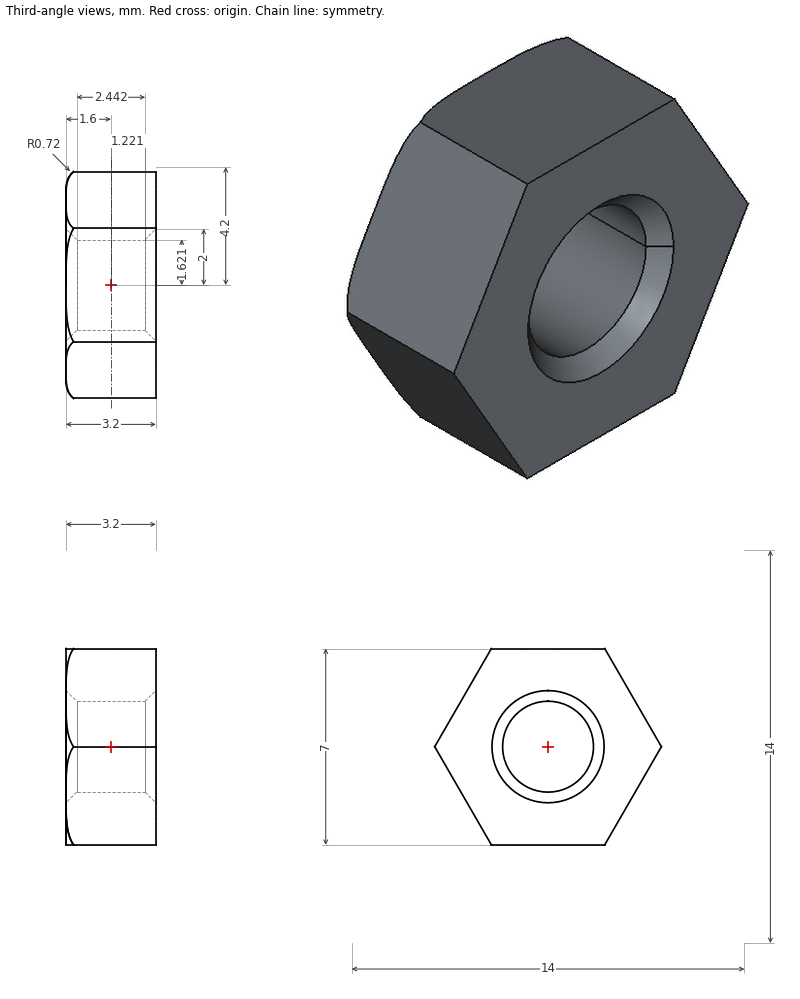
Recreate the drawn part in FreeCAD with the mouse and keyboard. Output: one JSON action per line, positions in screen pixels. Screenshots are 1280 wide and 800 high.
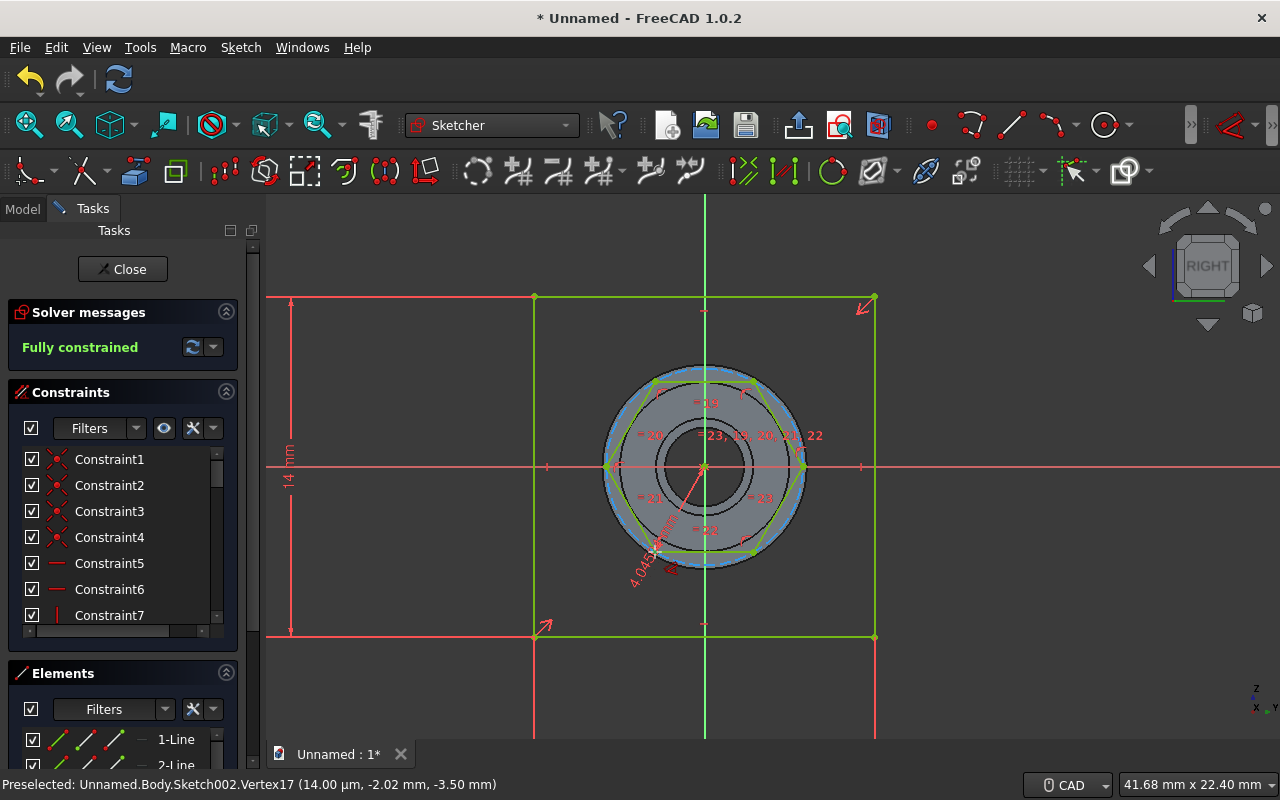
{"action": "left_click", "coordinate": [754, 382]}
{"action": "left_click", "coordinate": [812, 428]}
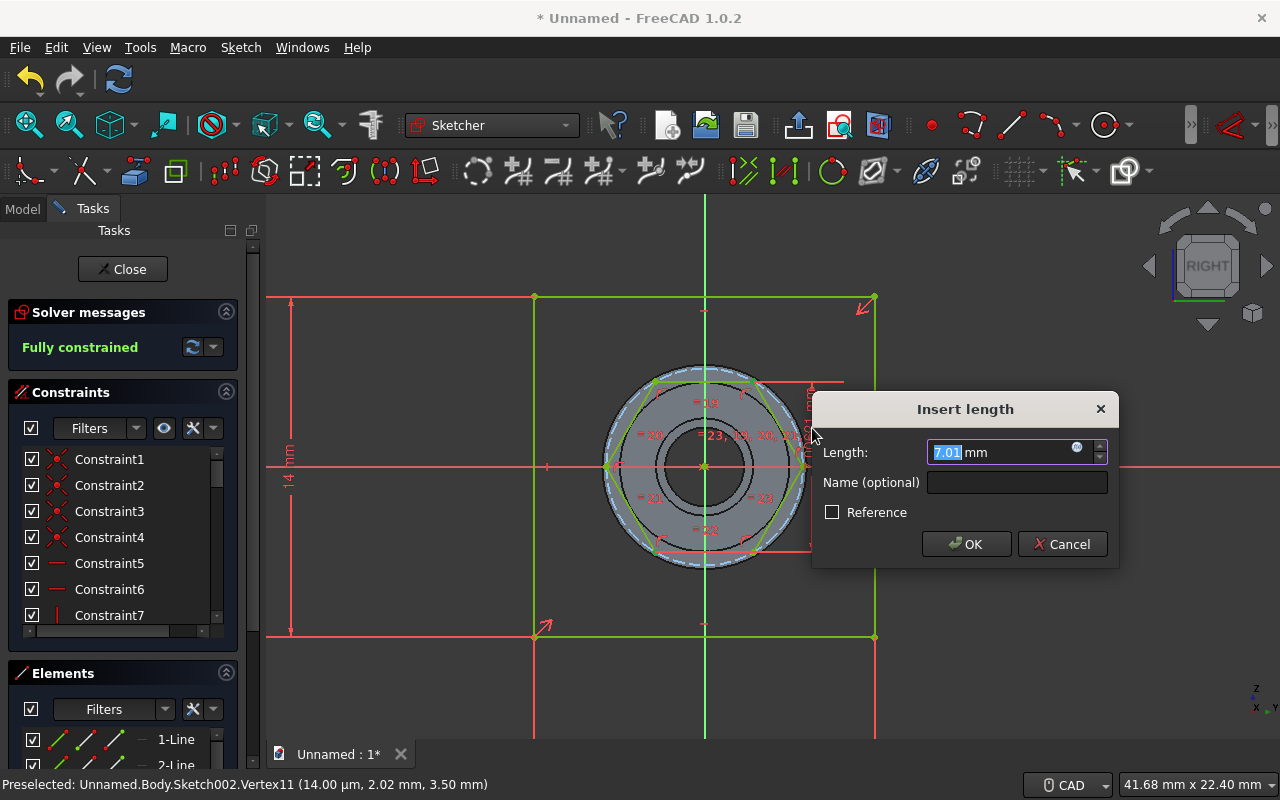
{"action": "type", "text": "7"}
{"action": "key", "text": "Return"}
{"action": "key", "text": "Escape"}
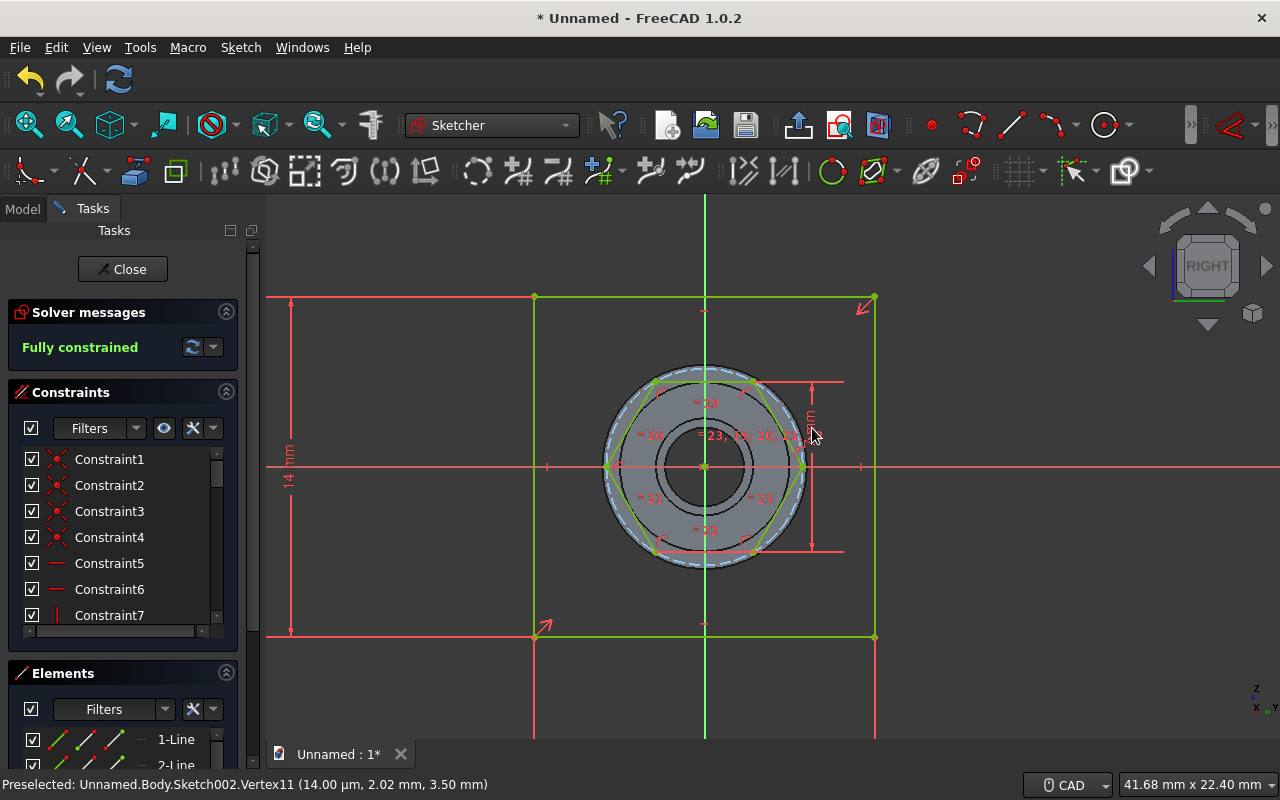
{"action": "left_click", "coordinate": [123, 269]}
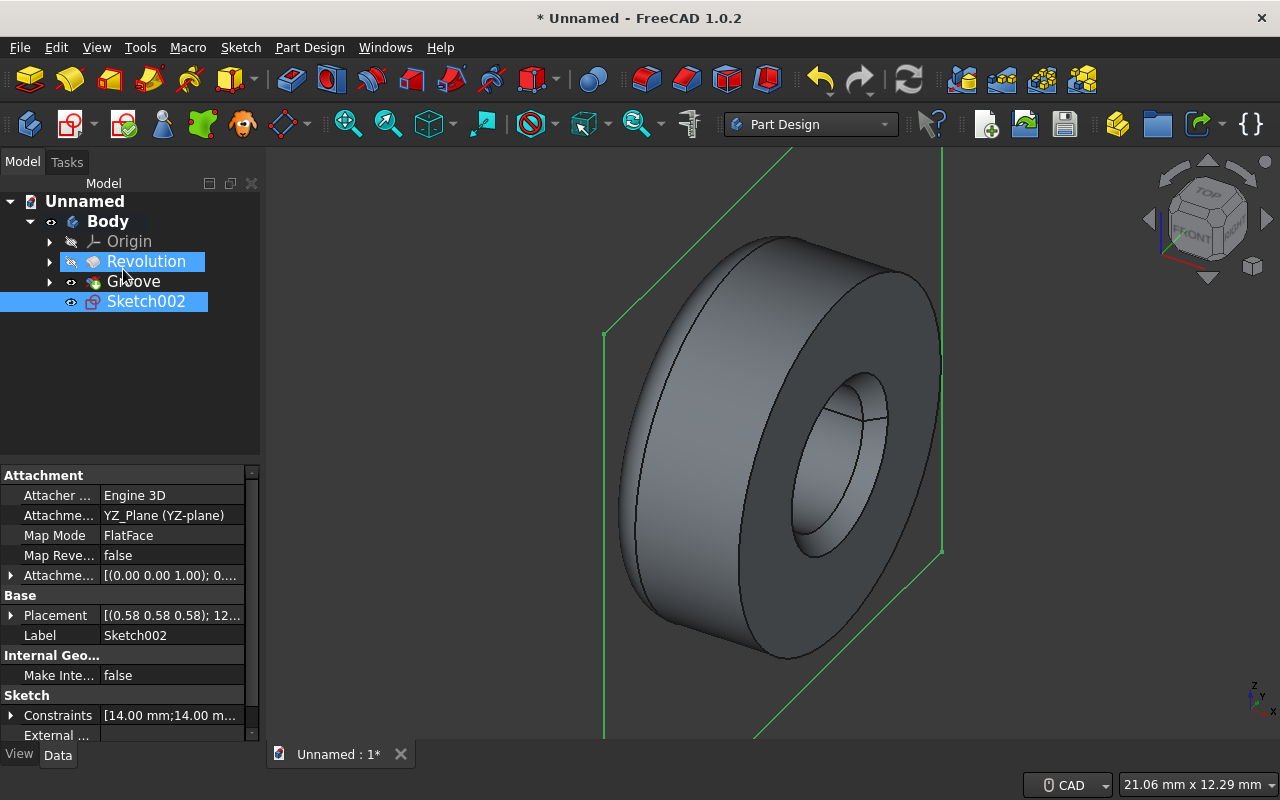
{"action": "left_click", "coordinate": [292, 80]}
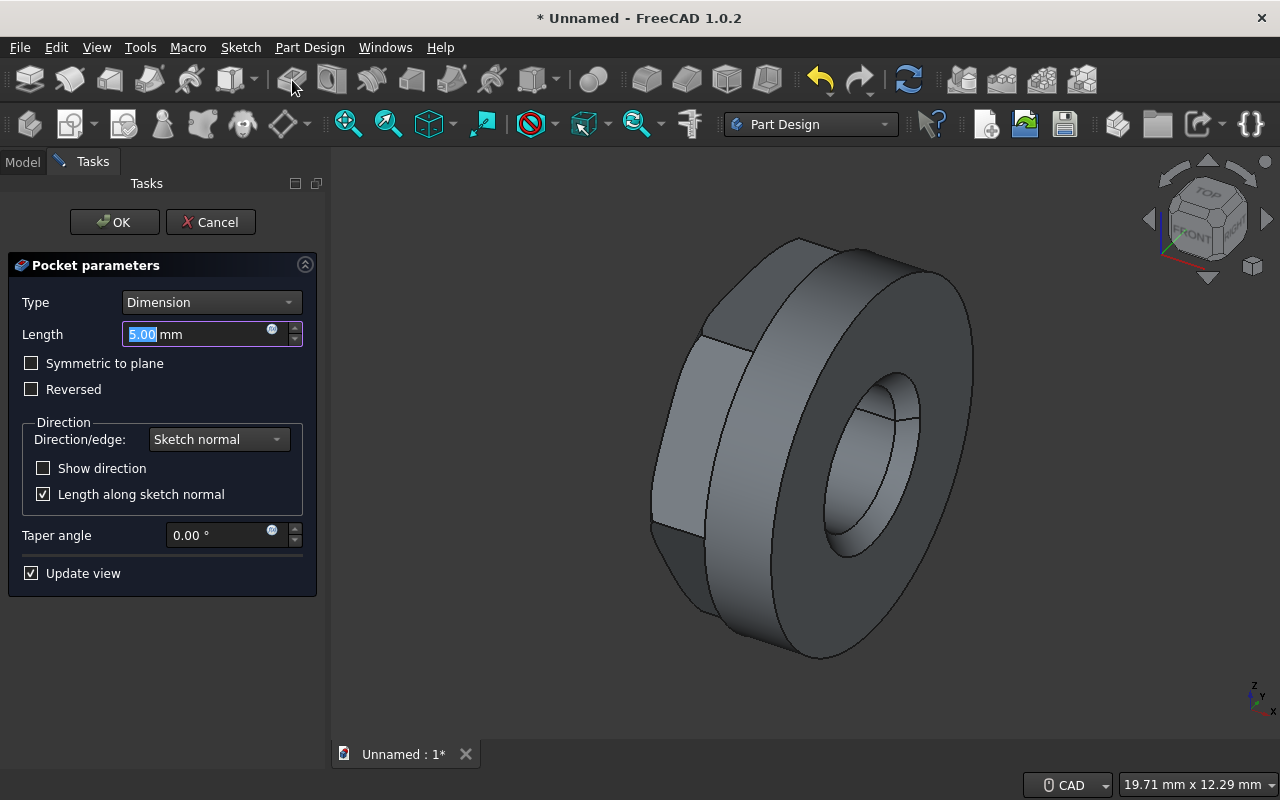
{"action": "type", "text": "3.2"}
{"action": "key", "text": "Tab"}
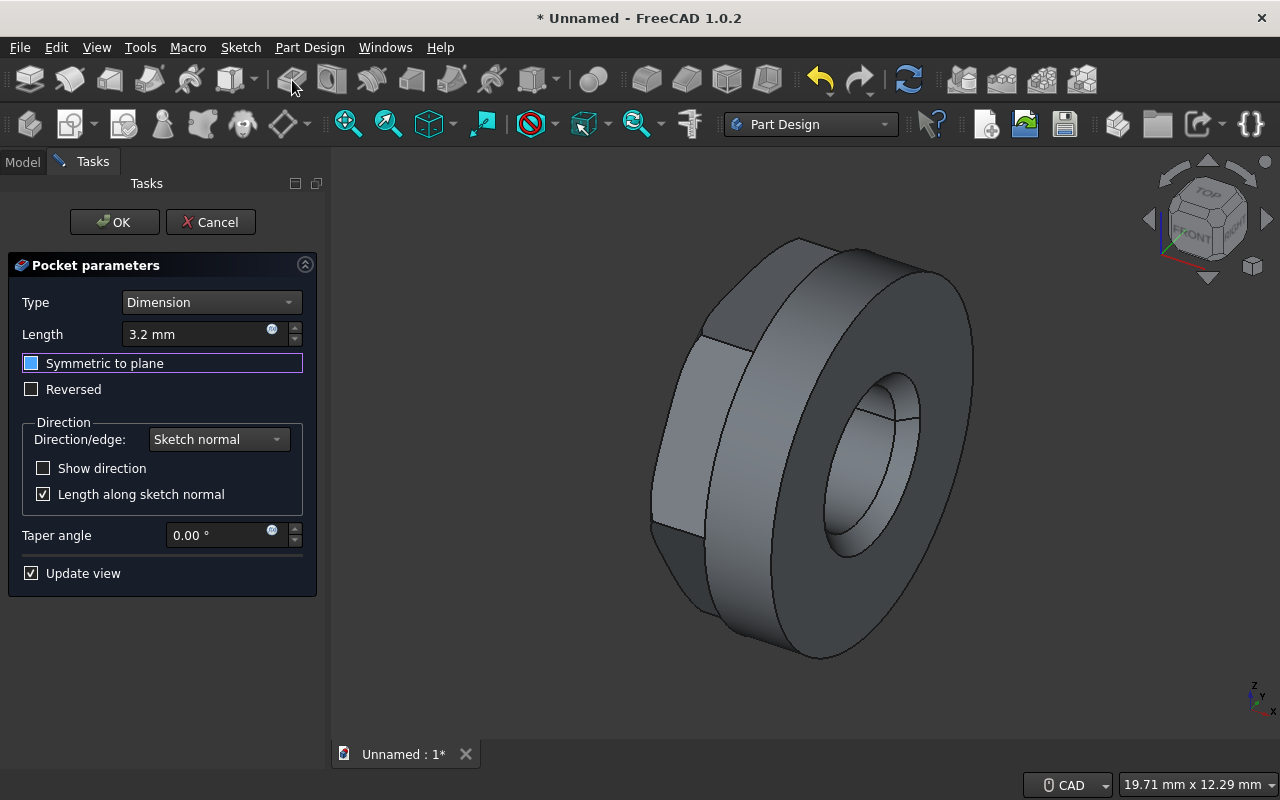
{"action": "left_click", "coordinate": [30, 363]}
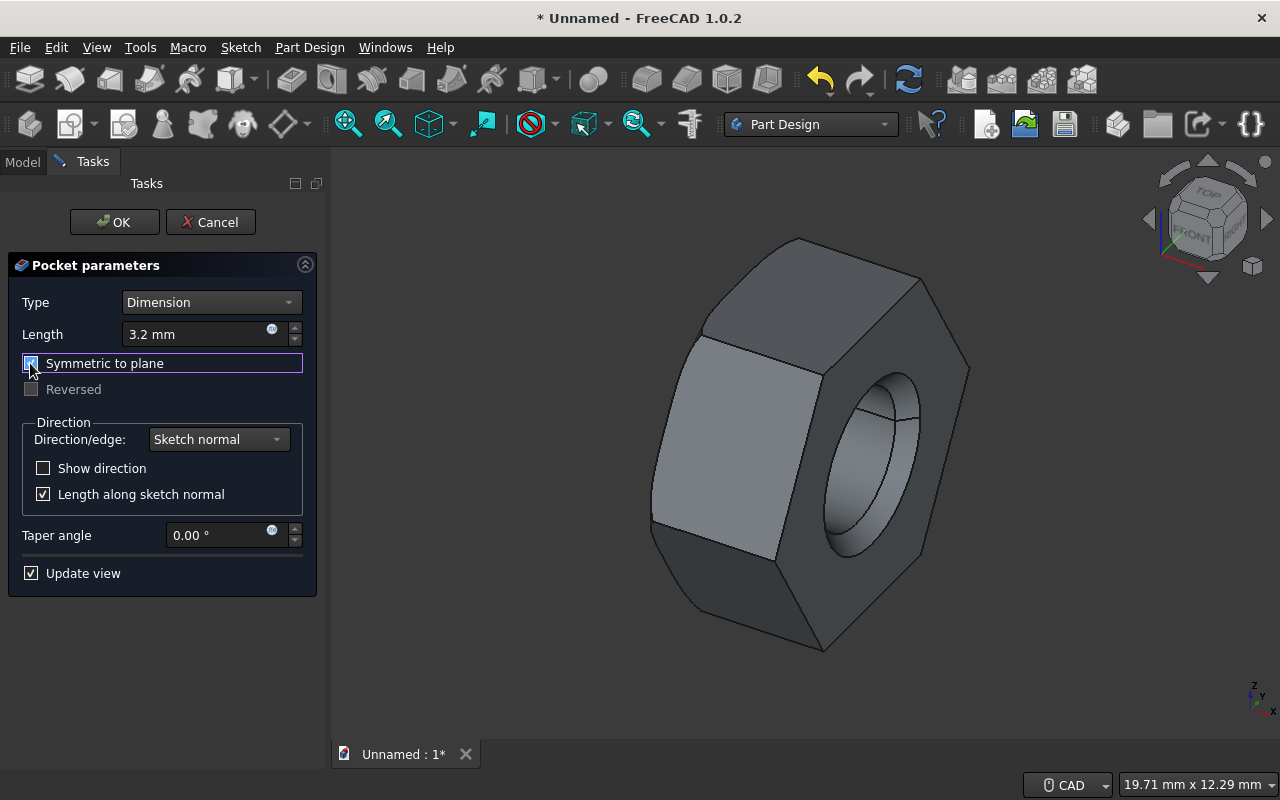
{"action": "left_click", "coordinate": [115, 222]}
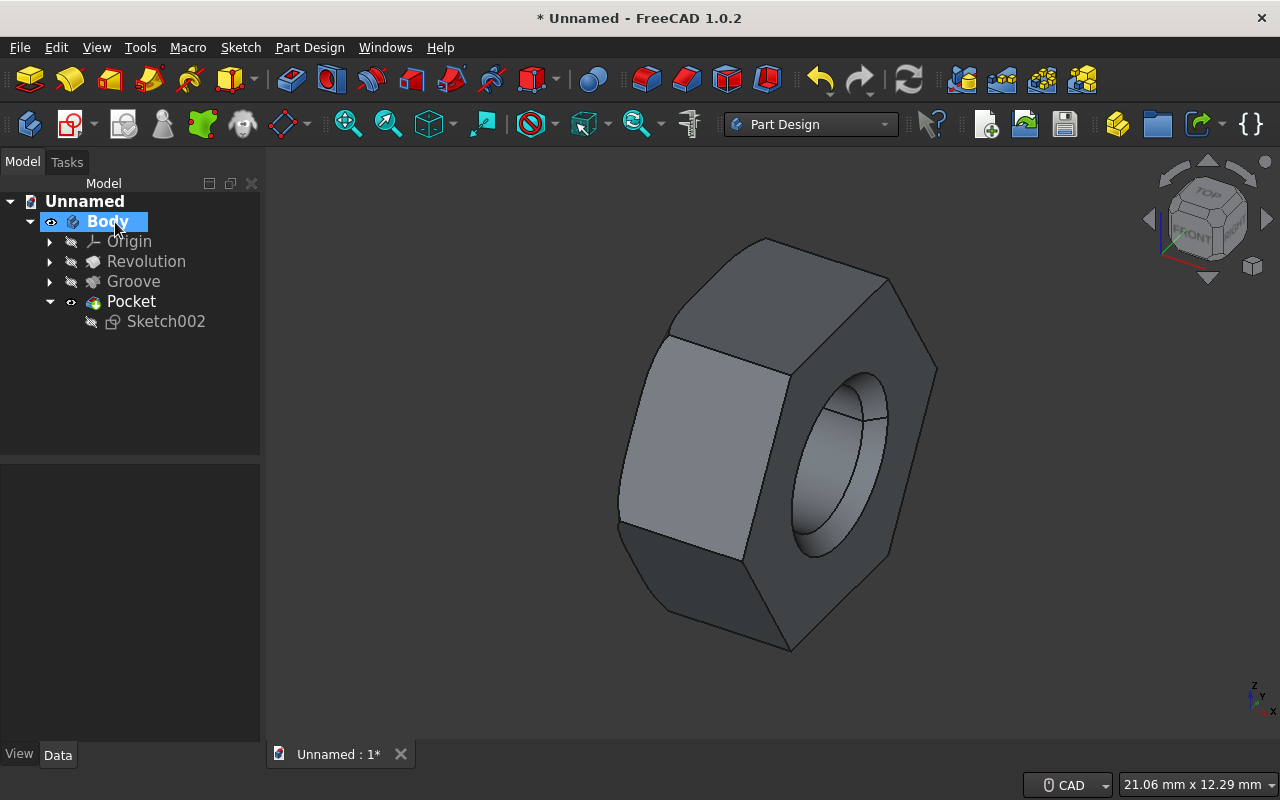
{"action": "key", "text": "0"}